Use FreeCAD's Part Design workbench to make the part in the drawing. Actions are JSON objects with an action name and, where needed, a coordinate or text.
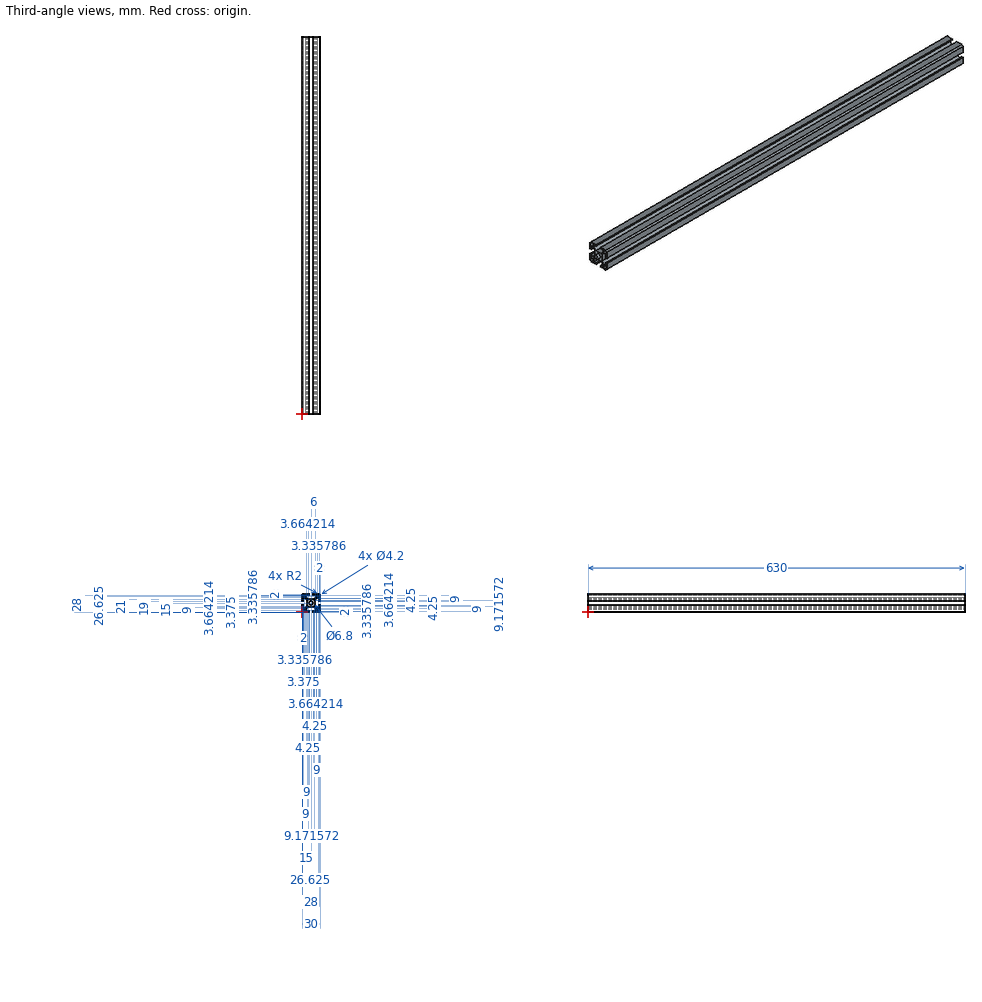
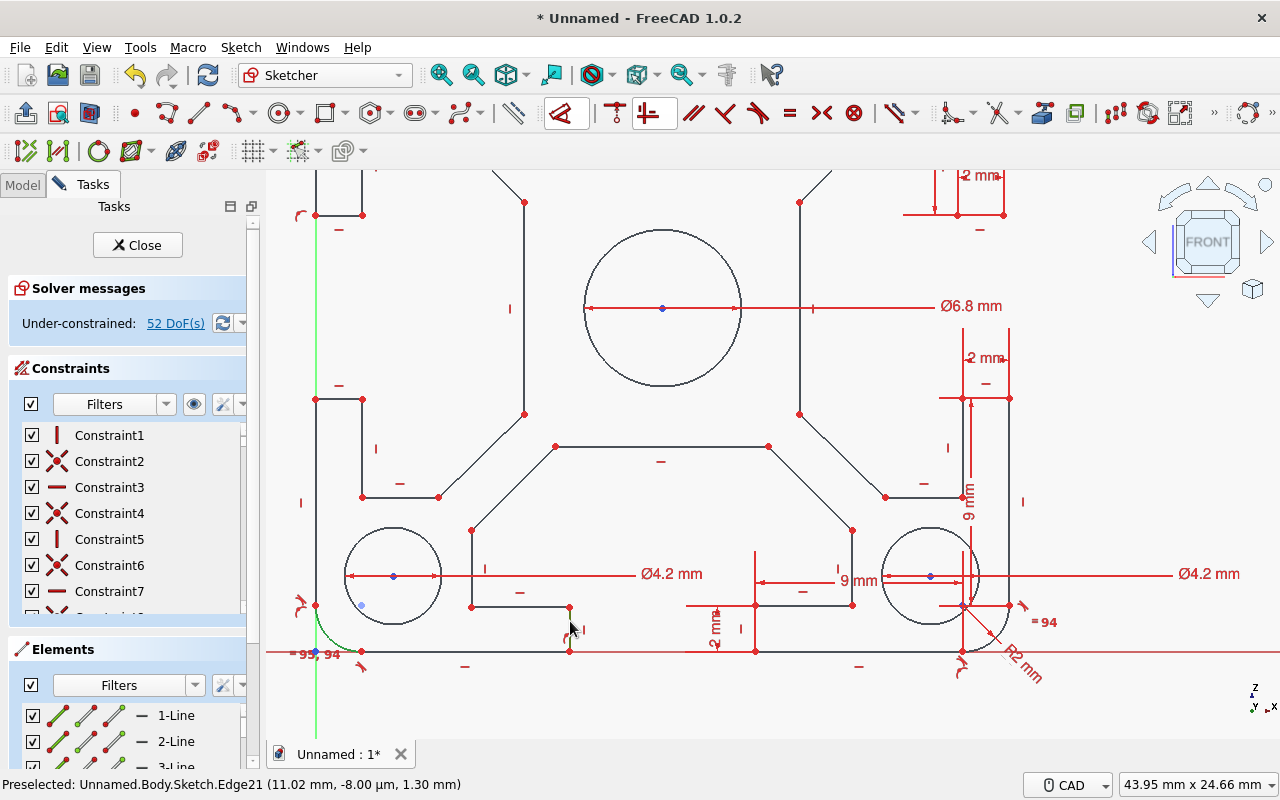
{"action": "left_click", "coordinate": [584, 114]}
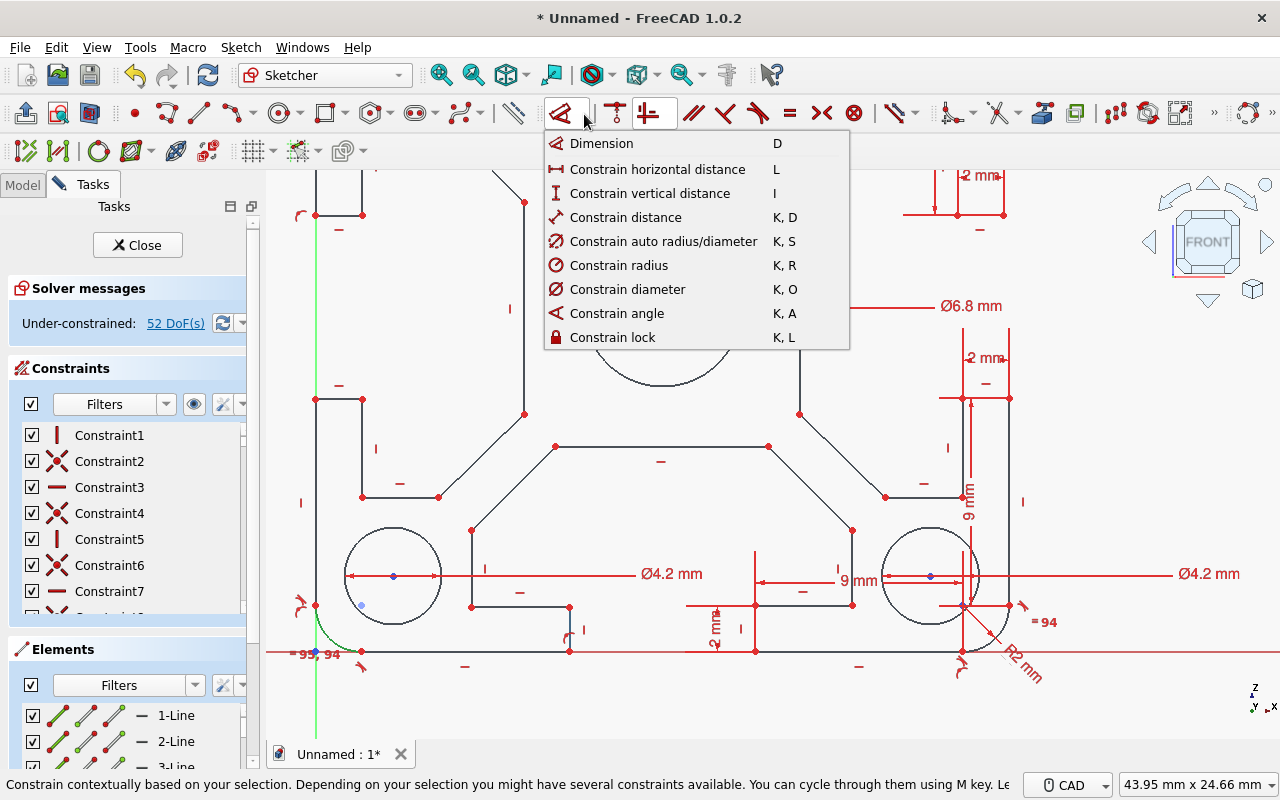
{"action": "left_click", "coordinate": [697, 193]}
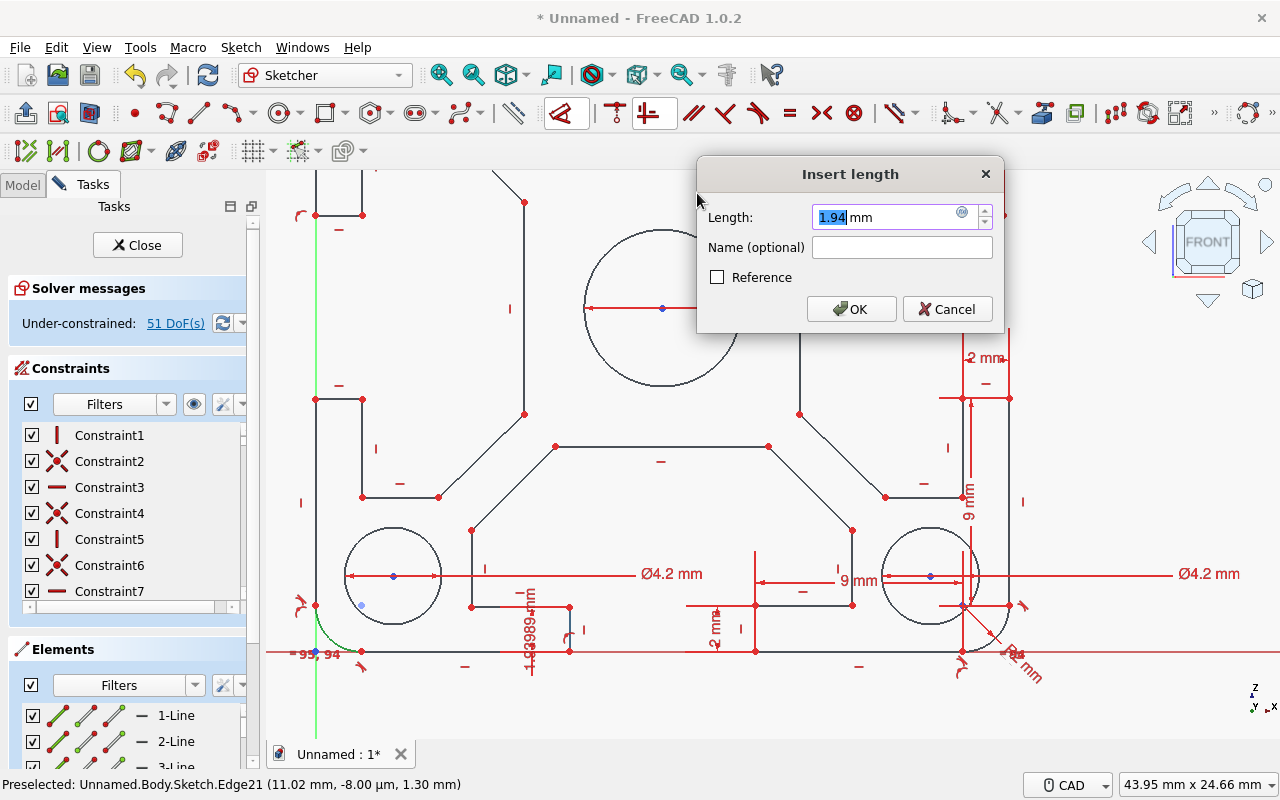
{"action": "type", "text": "2"}
{"action": "key", "text": "Return"}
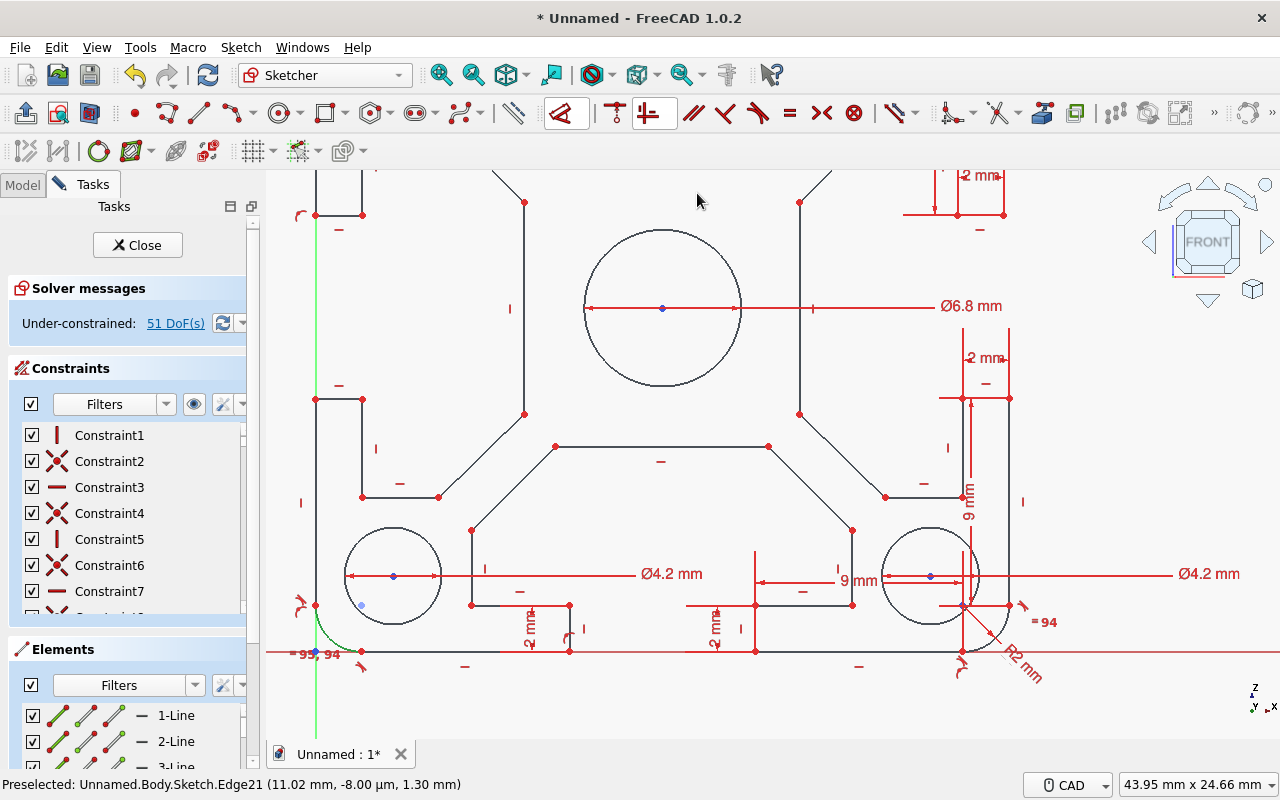
{"action": "left_click", "coordinate": [508, 652]}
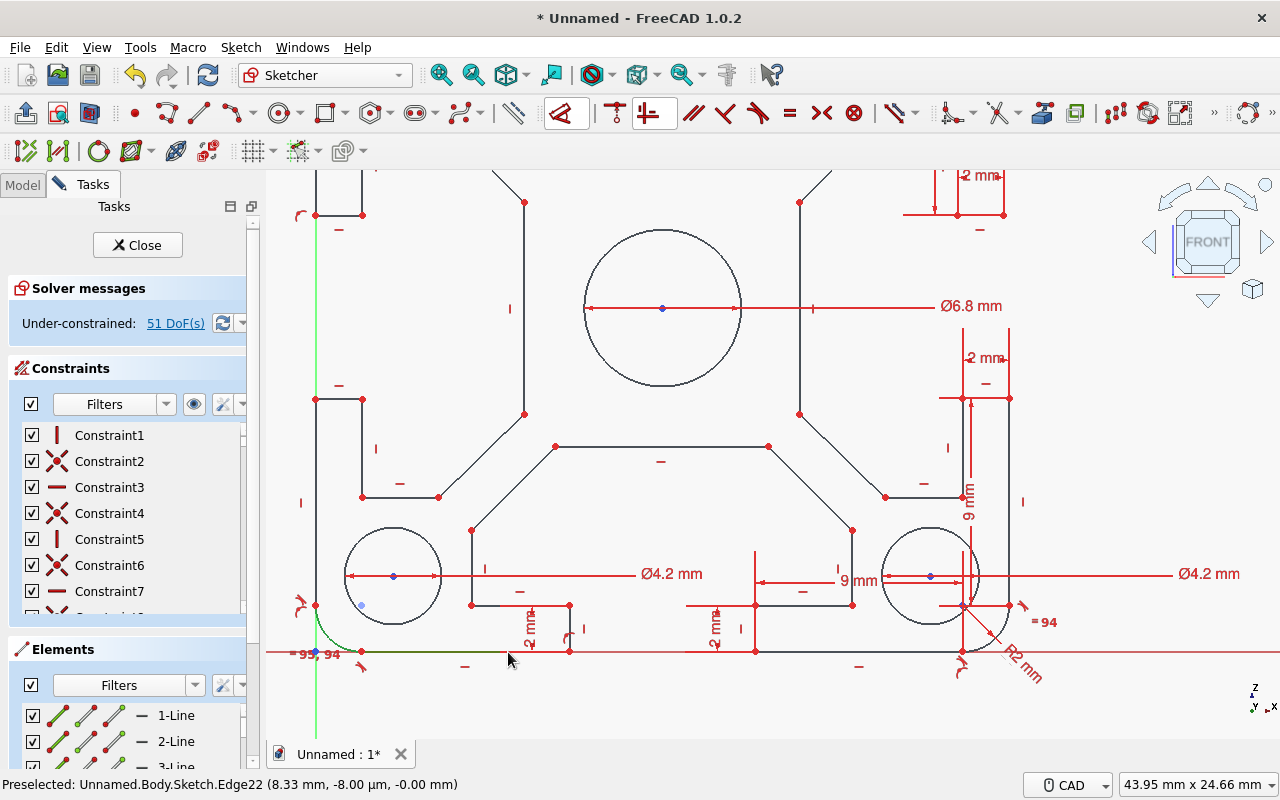
{"action": "left_click", "coordinate": [584, 114]}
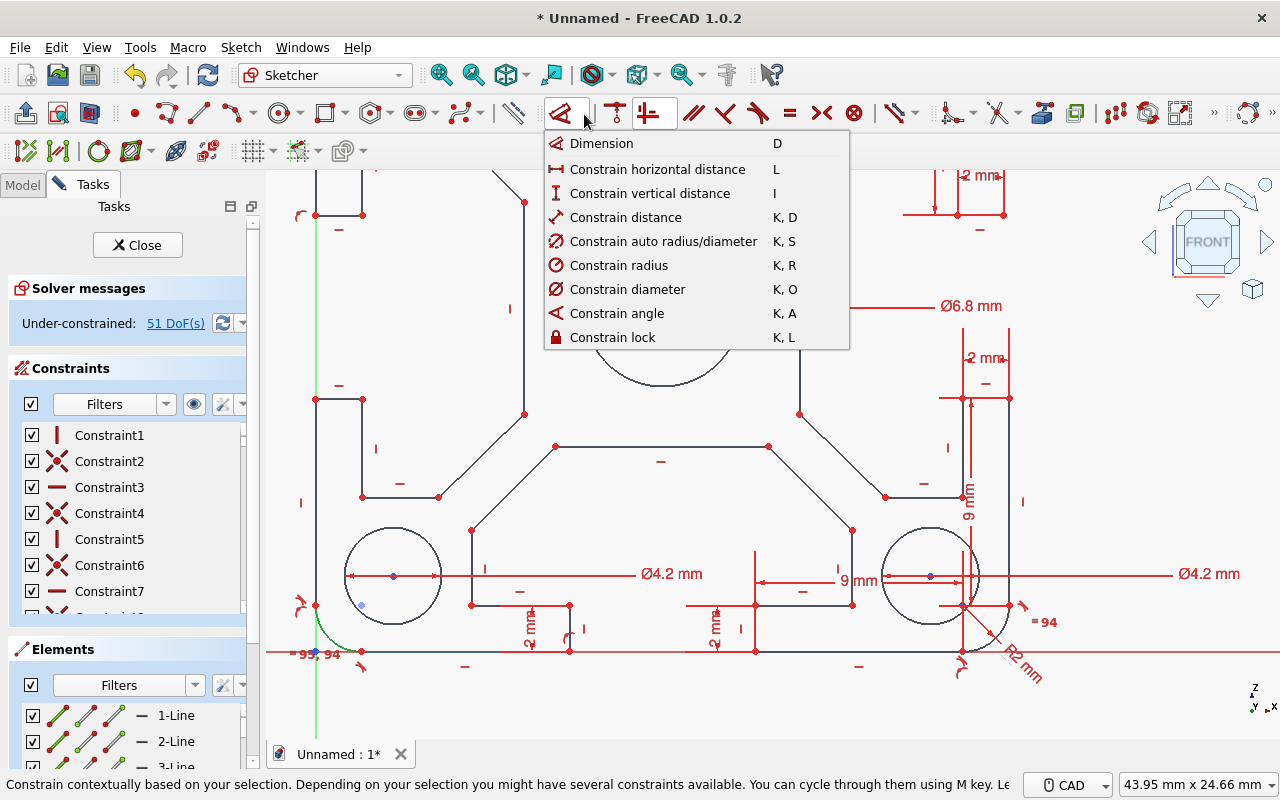
{"action": "left_click", "coordinate": [697, 169]}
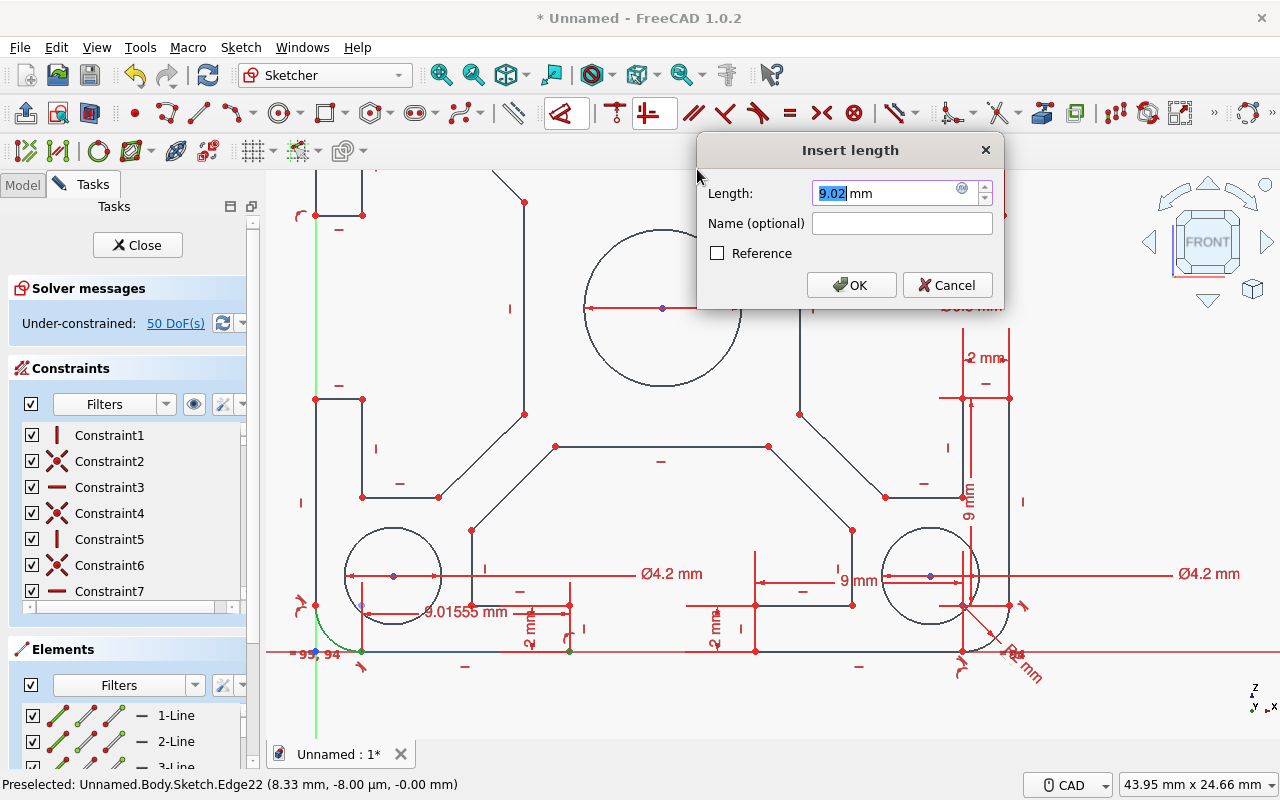
{"action": "type", "text": "9"}
{"action": "key", "text": "Return"}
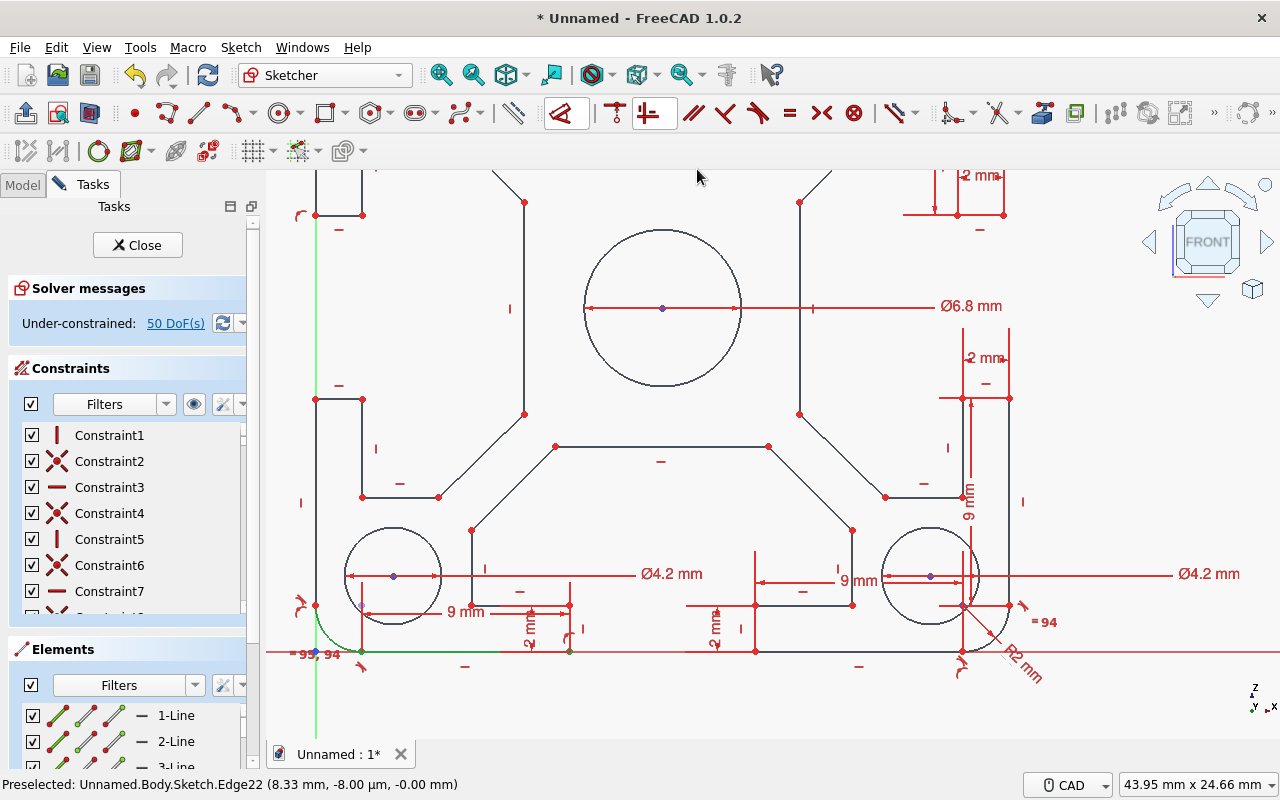
{"action": "left_click", "coordinate": [316, 544]}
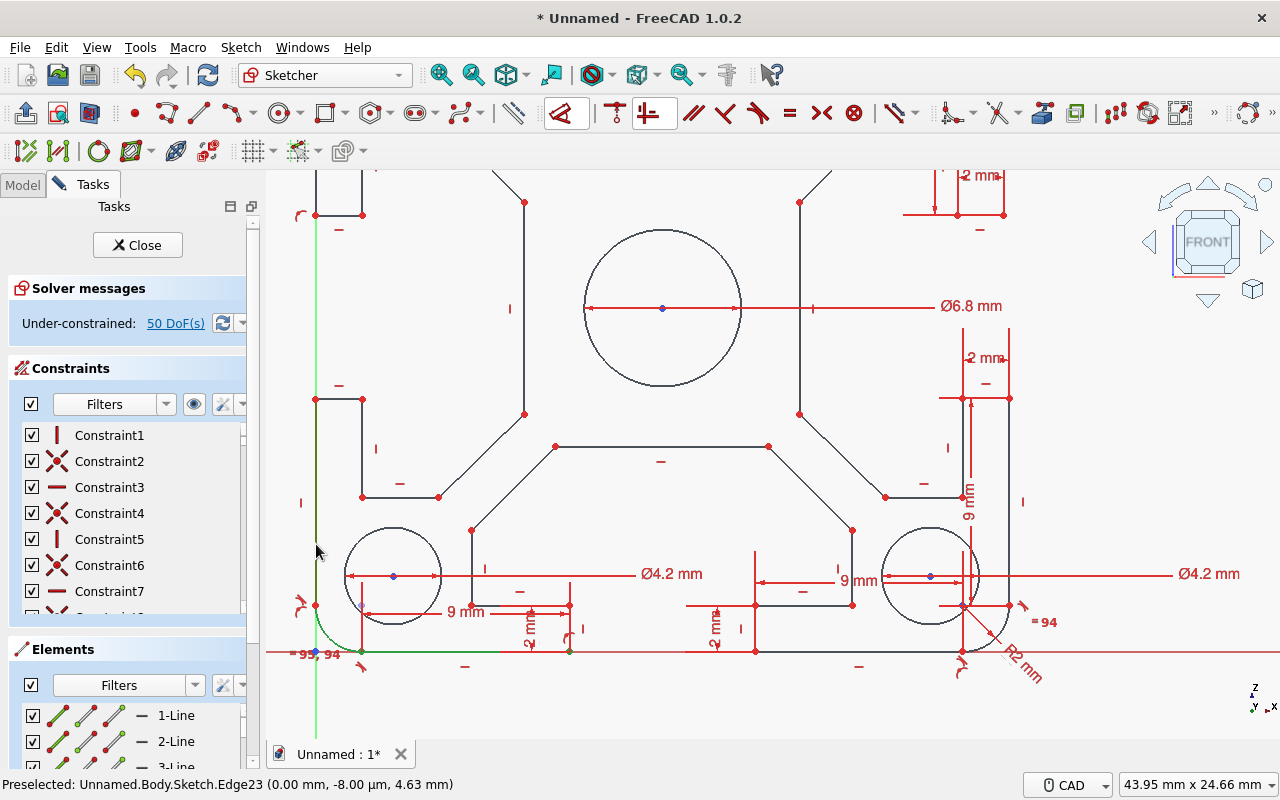
{"action": "left_click", "coordinate": [584, 114]}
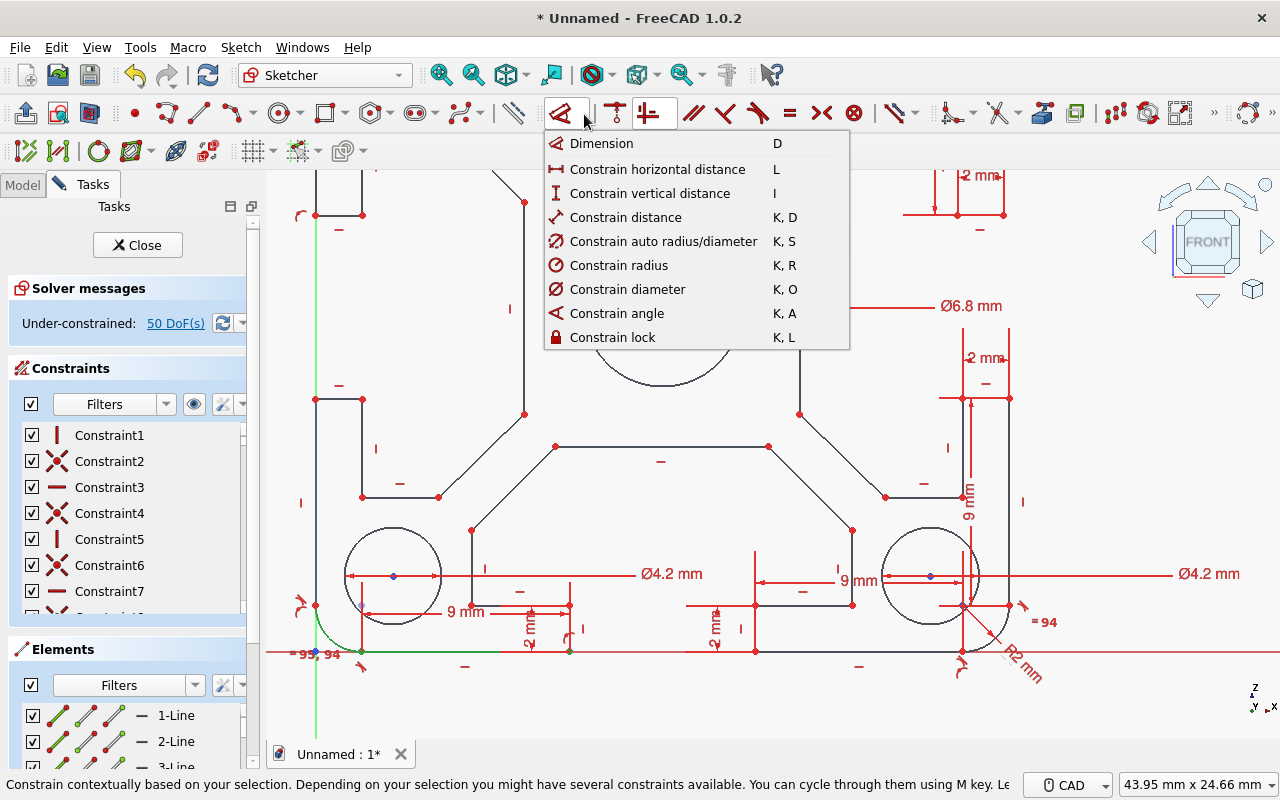
{"action": "left_click", "coordinate": [697, 193]}